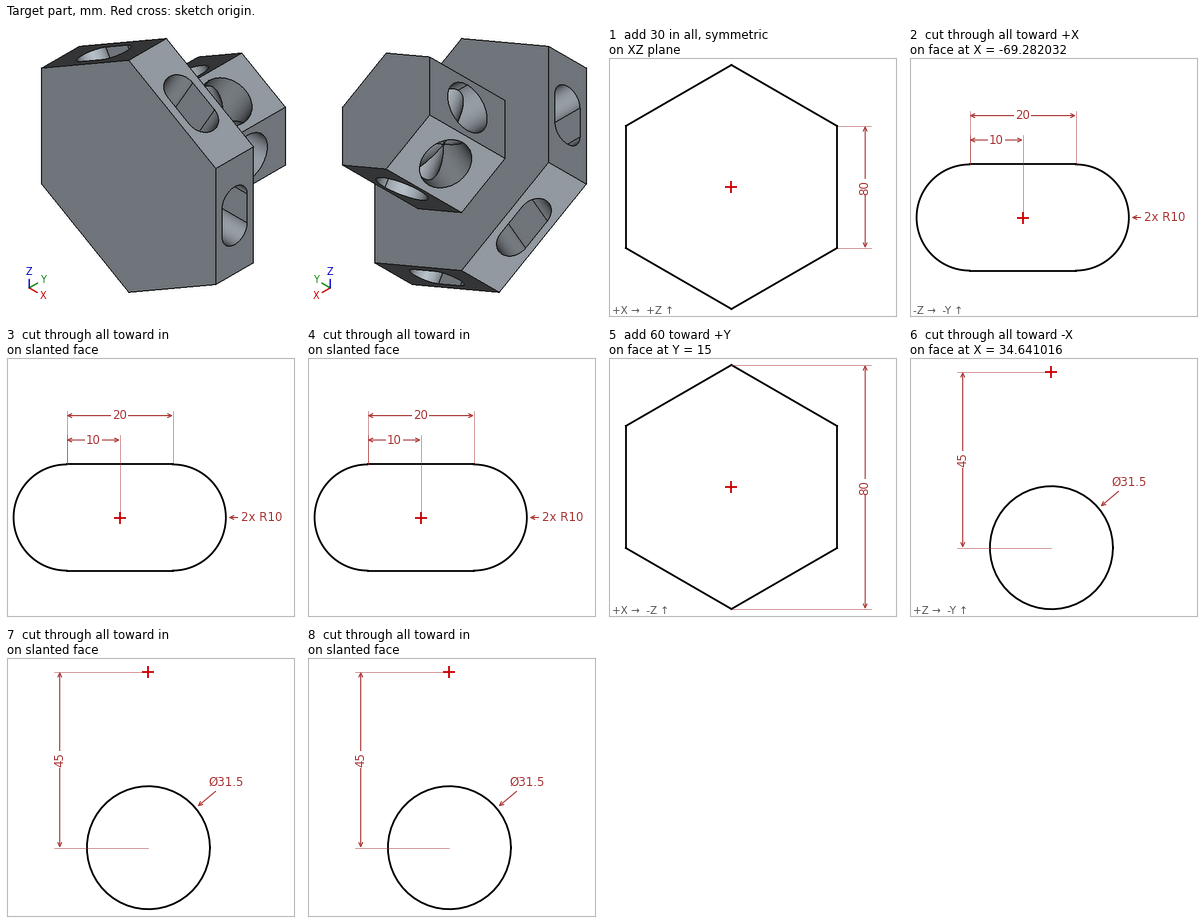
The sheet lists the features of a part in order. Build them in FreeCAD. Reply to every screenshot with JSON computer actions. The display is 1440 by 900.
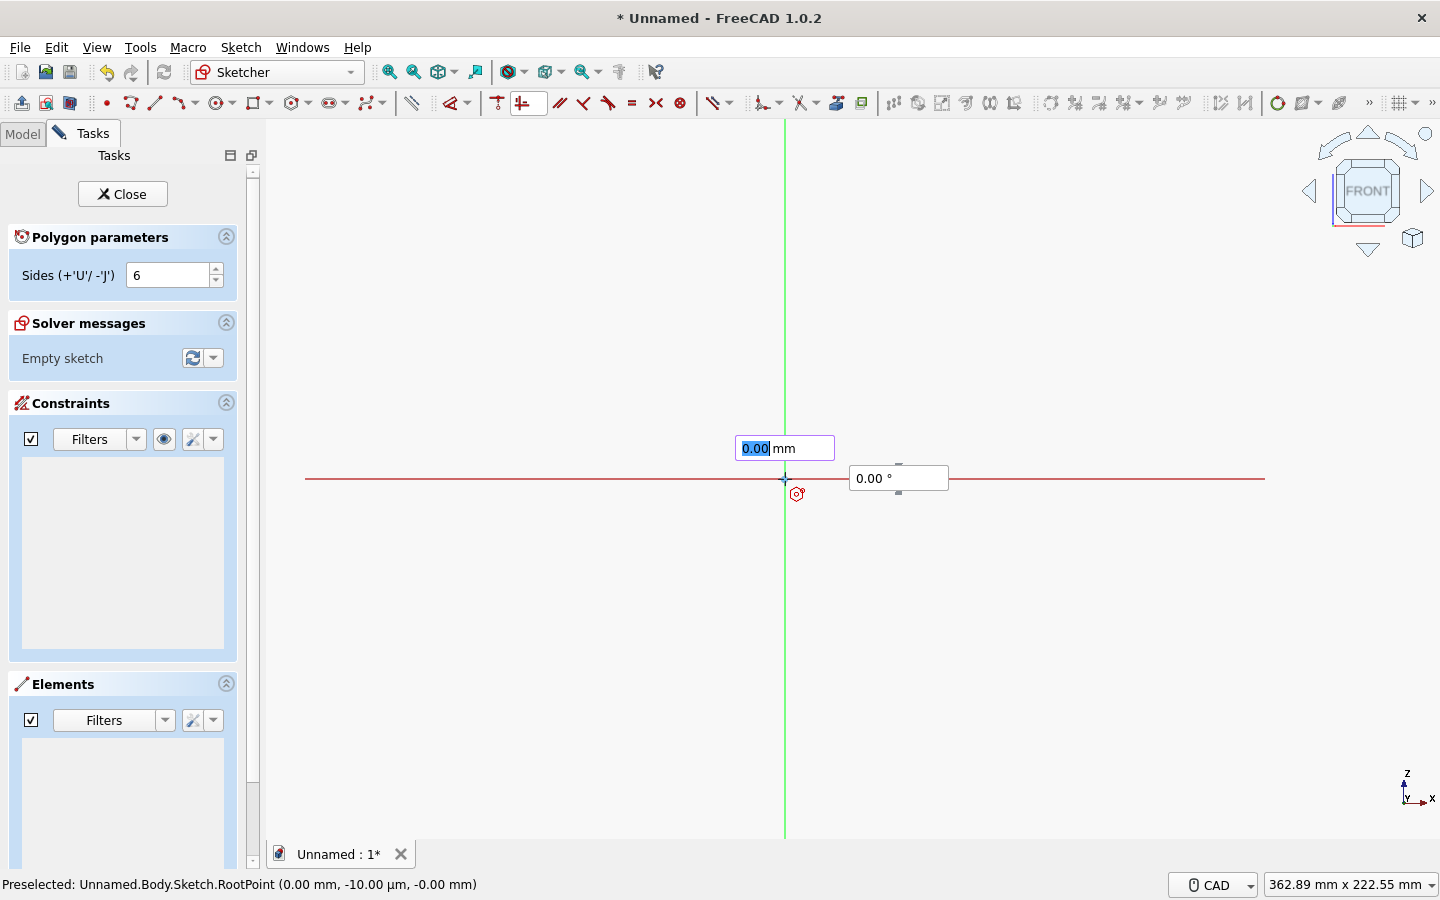
{"action": "left_click", "coordinate": [785, 738]}
{"action": "right_click", "coordinate": [785, 738]}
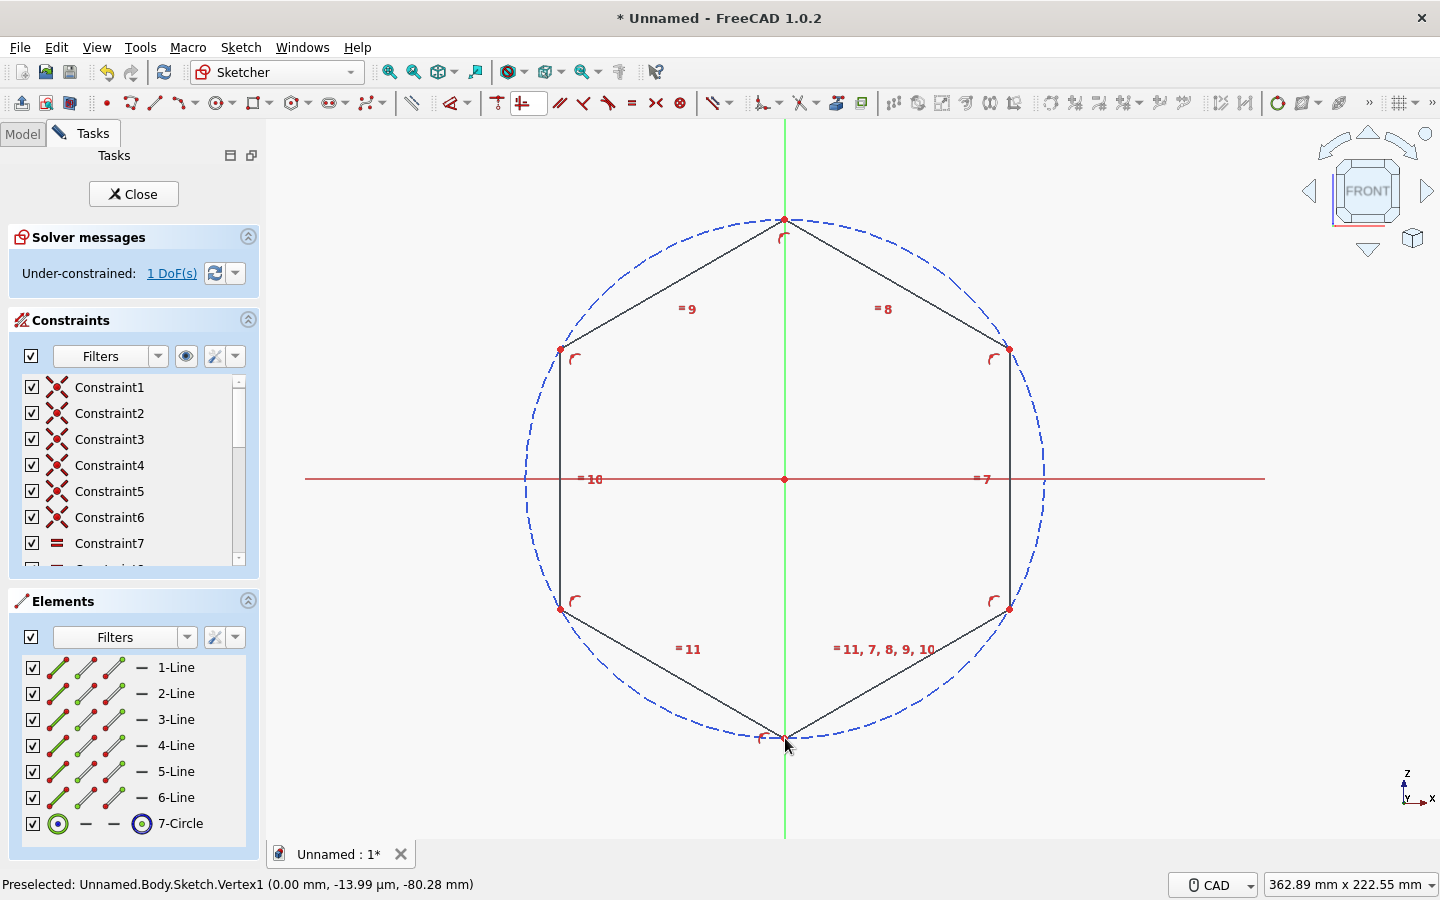
{"action": "left_click", "coordinate": [1010, 531]}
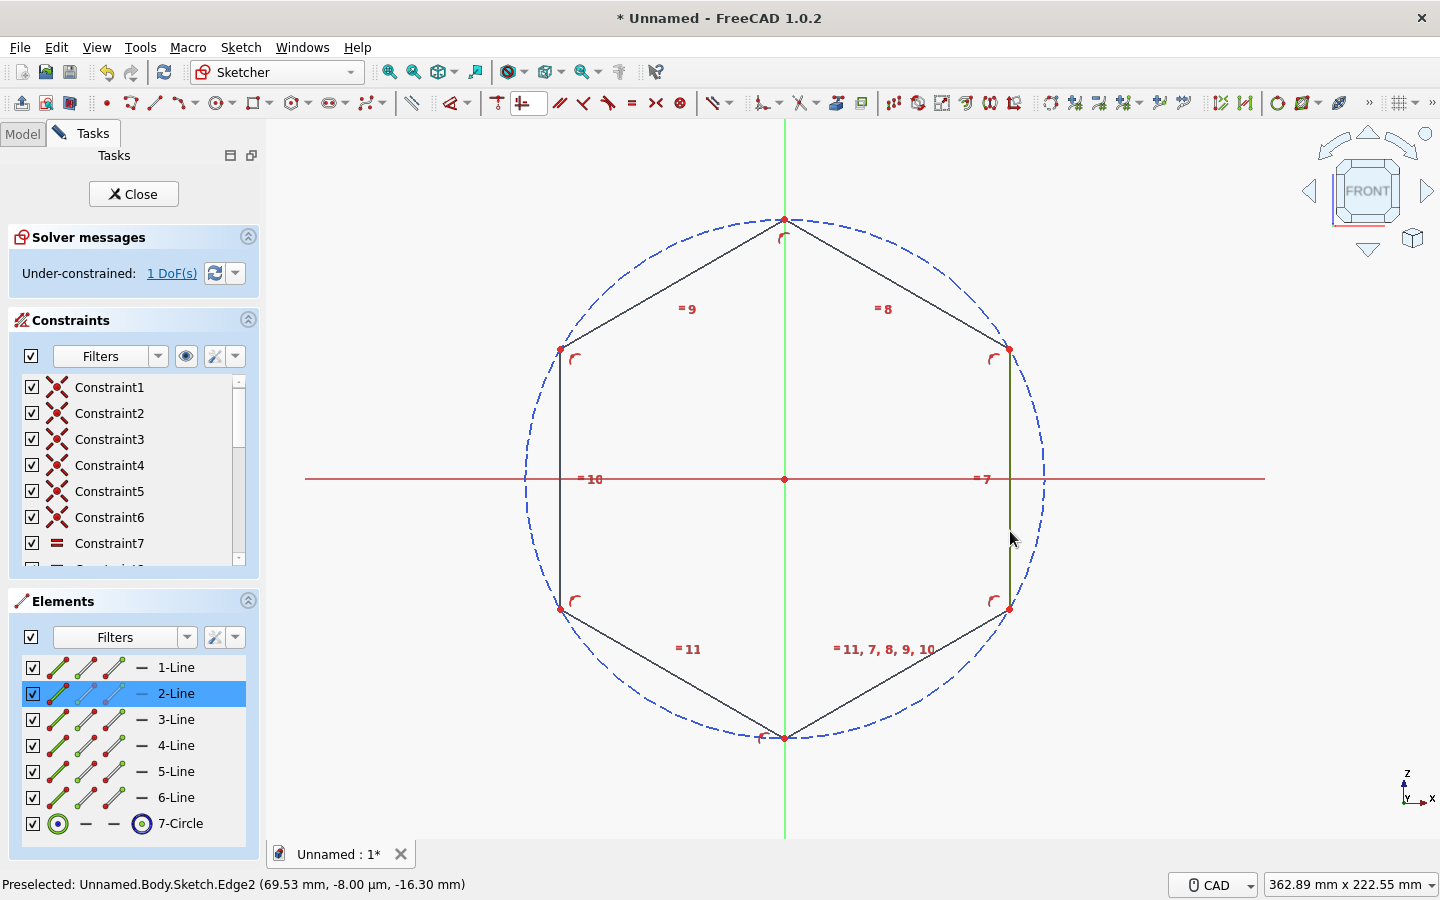
{"action": "left_click", "coordinate": [470, 104]}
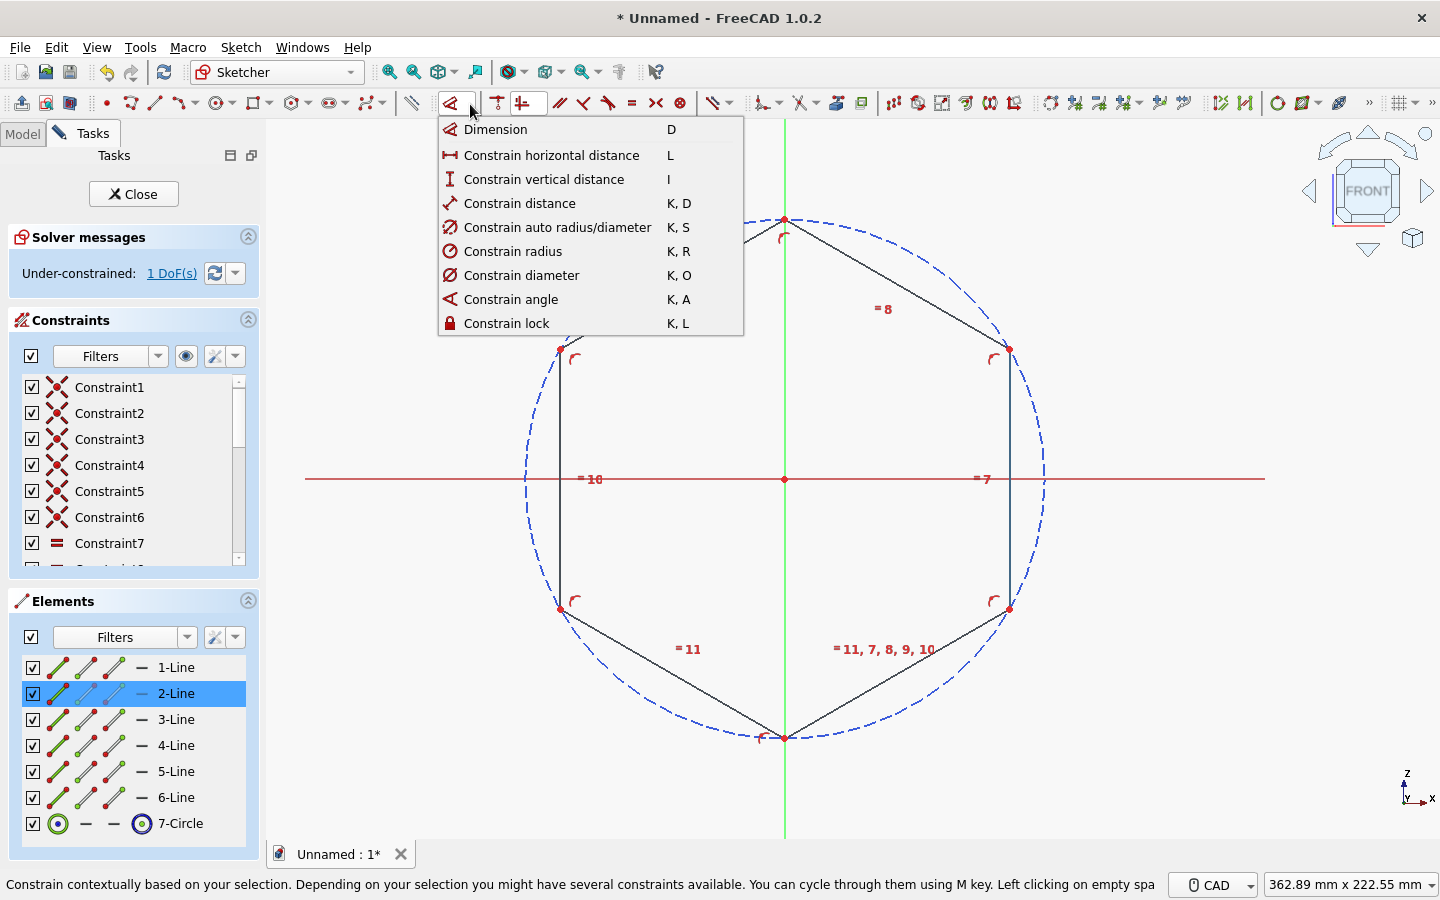
{"action": "left_click", "coordinate": [591, 179]}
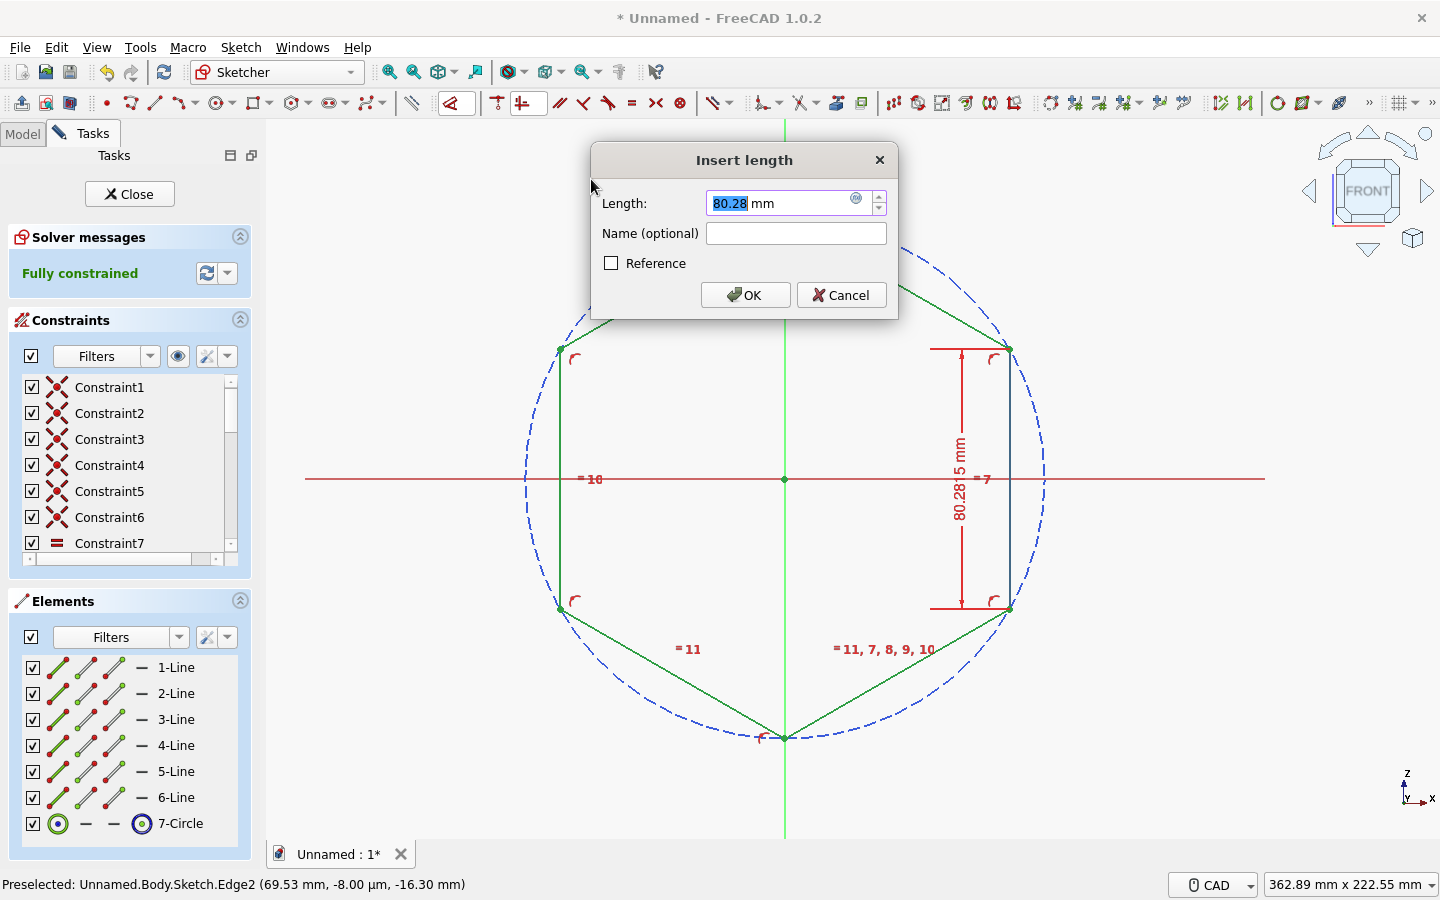
{"action": "type", "text": "80"}
{"action": "key", "text": "Return"}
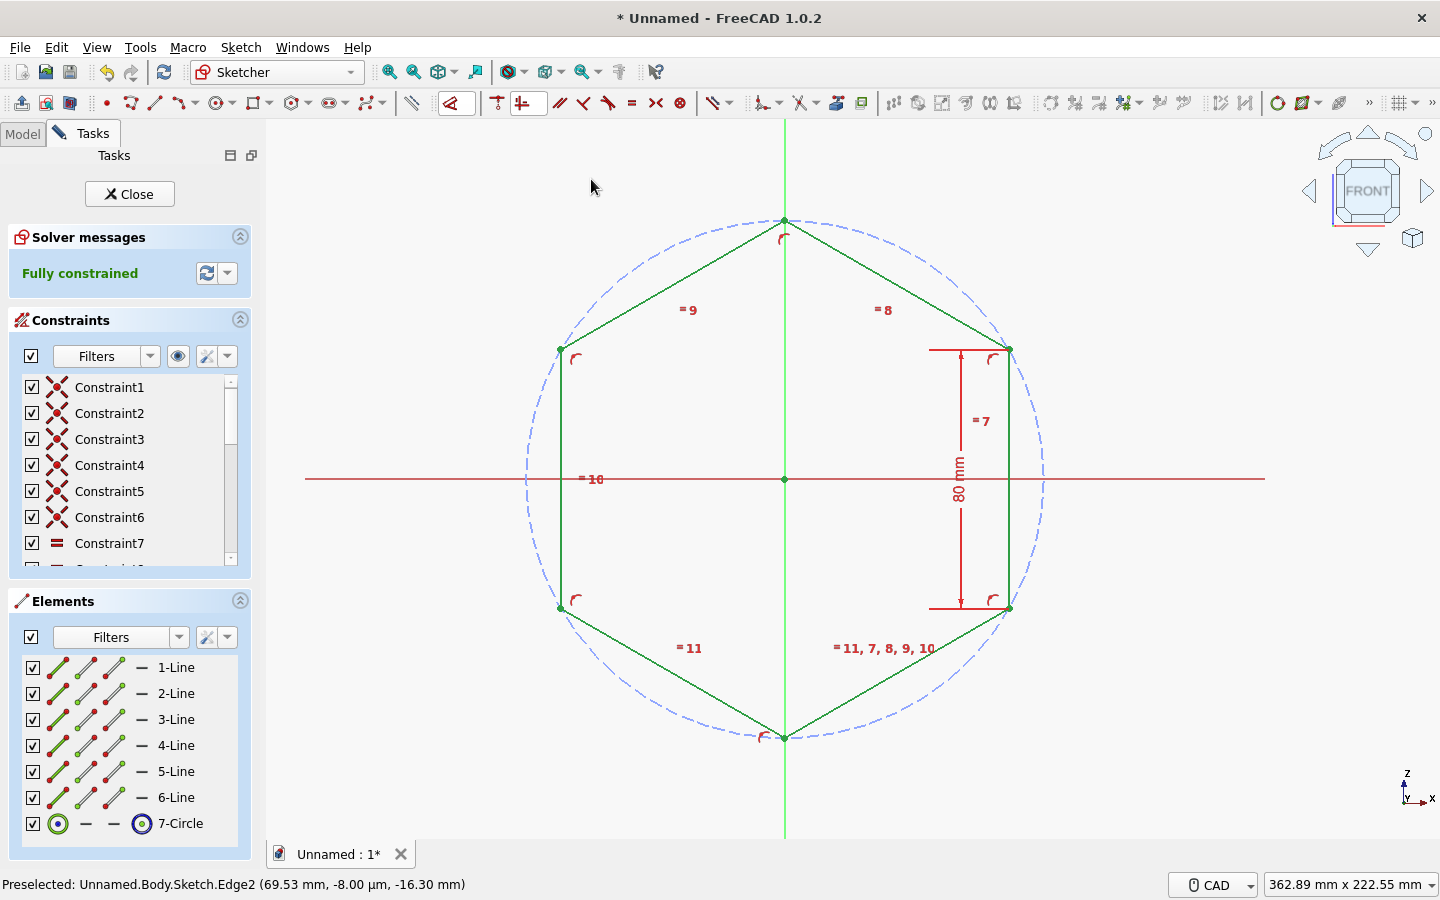
{"action": "left_click", "coordinate": [130, 194]}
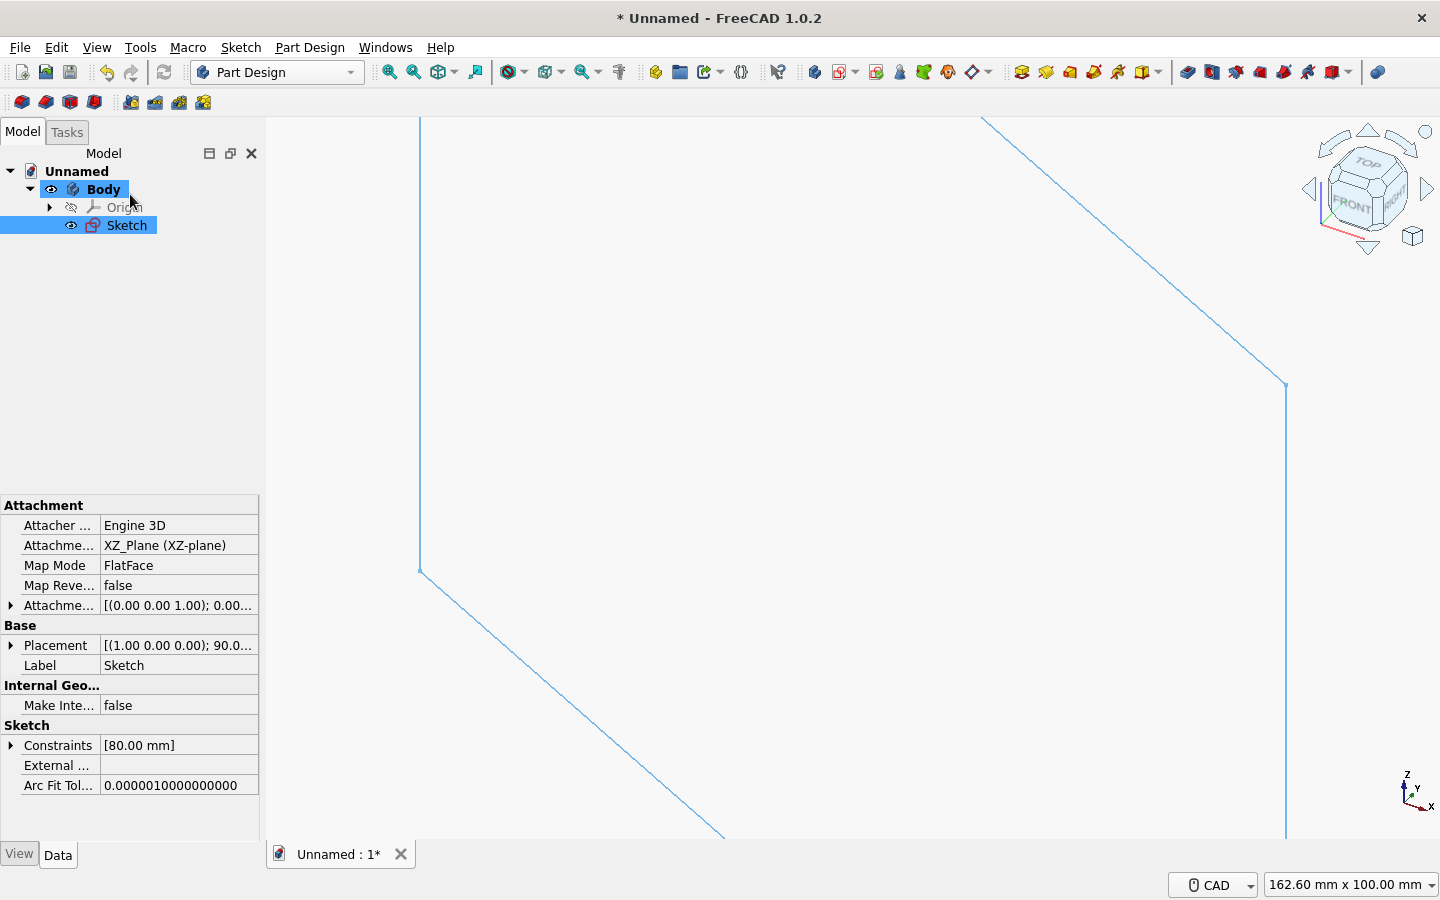
{"action": "left_click", "coordinate": [1022, 72]}